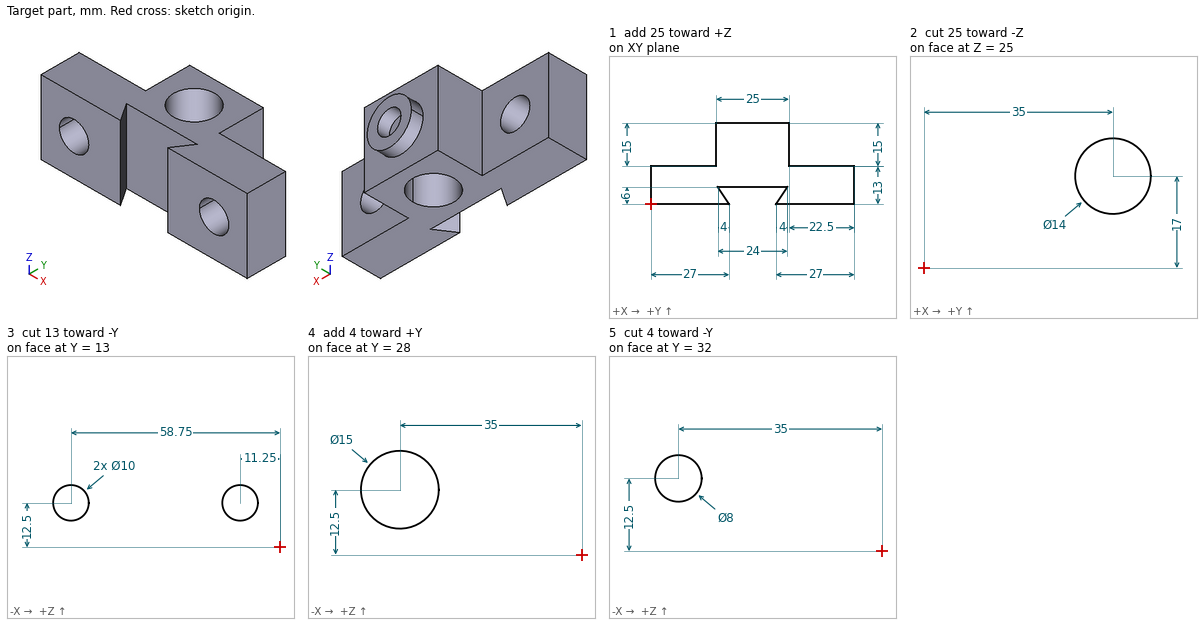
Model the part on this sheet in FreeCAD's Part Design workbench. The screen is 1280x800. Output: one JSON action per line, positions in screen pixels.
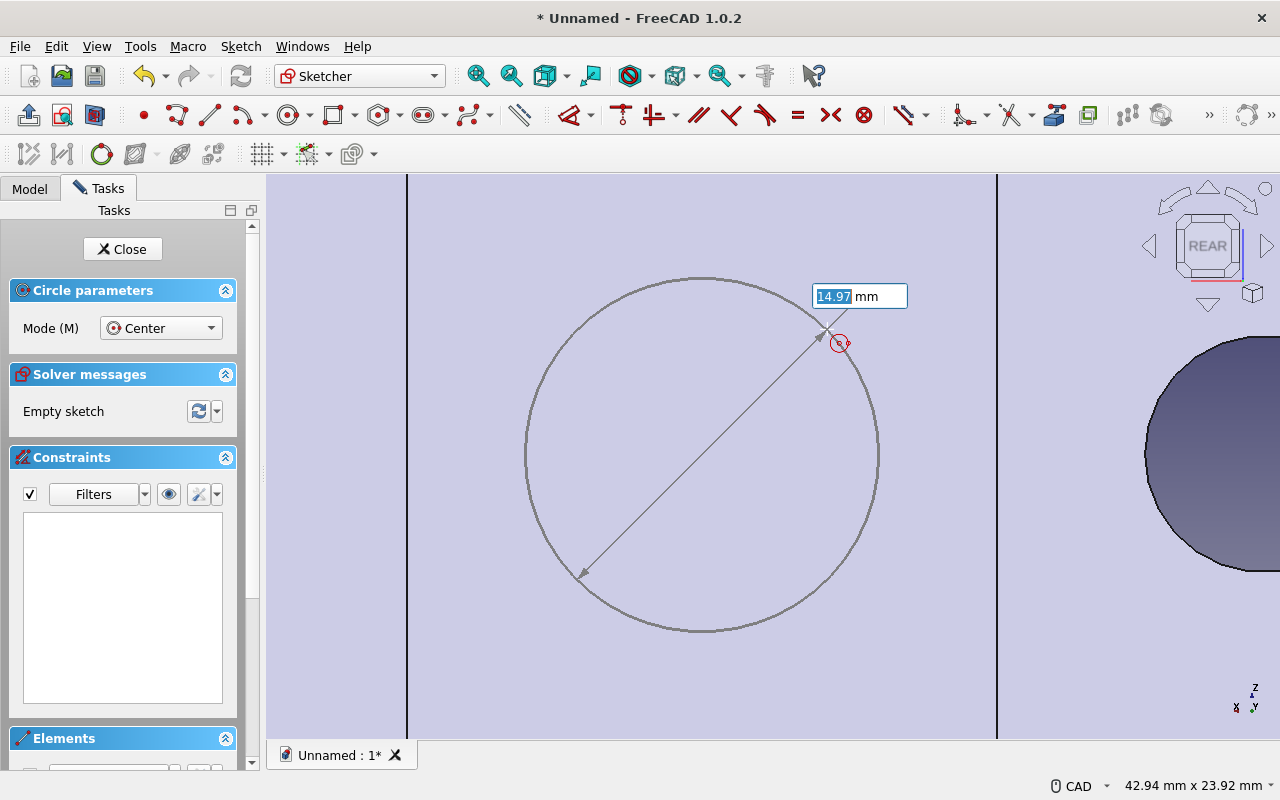
{"action": "type", "text": "15"}
{"action": "key", "text": "Return"}
{"action": "key", "text": "Escape"}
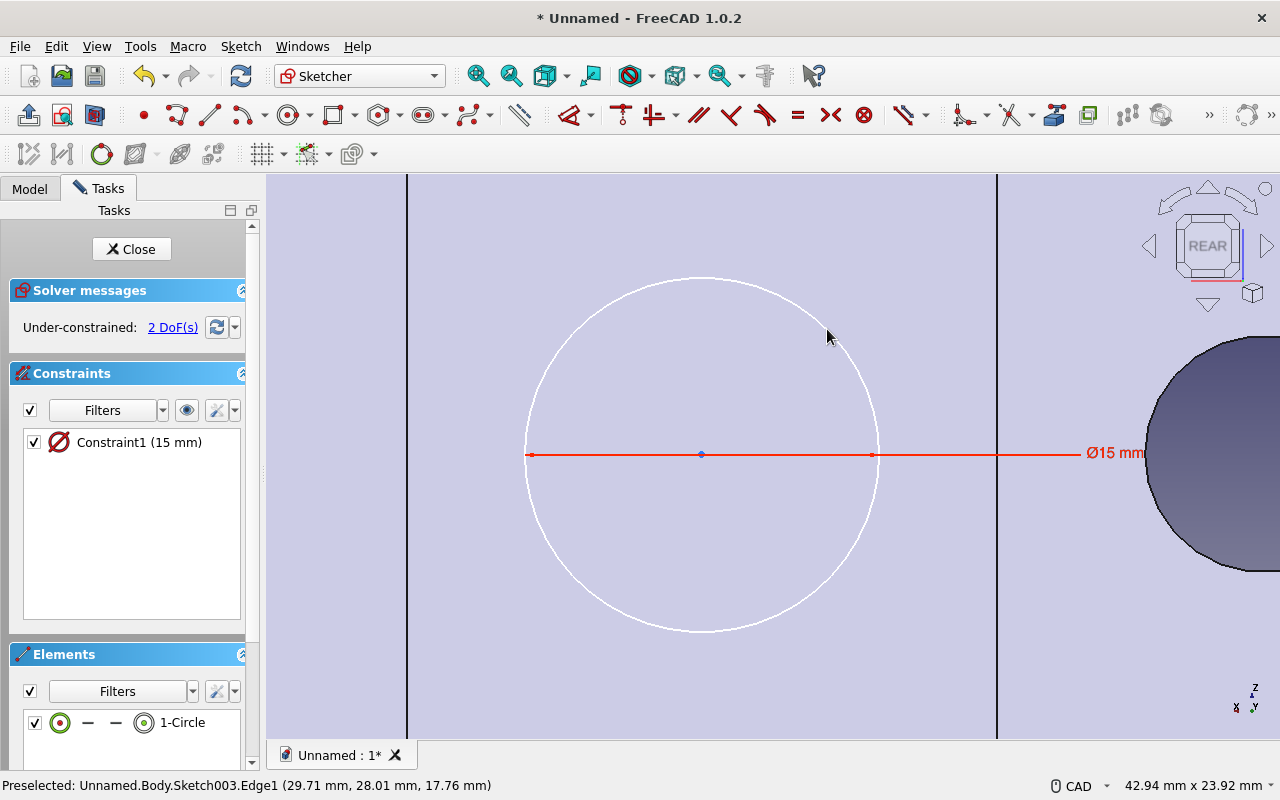
{"action": "left_click", "coordinate": [568, 116]}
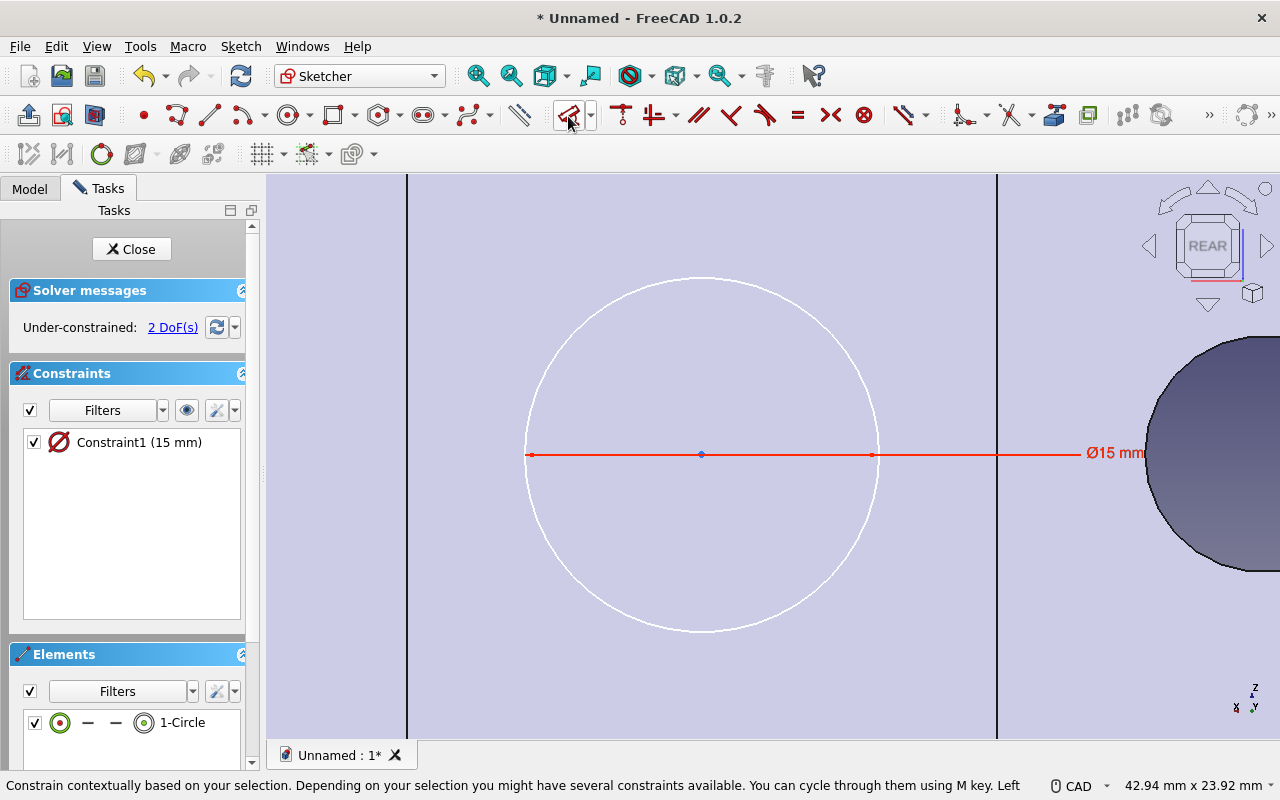
{"action": "left_click", "coordinate": [702, 455]}
{"action": "left_click", "coordinate": [908, 421]}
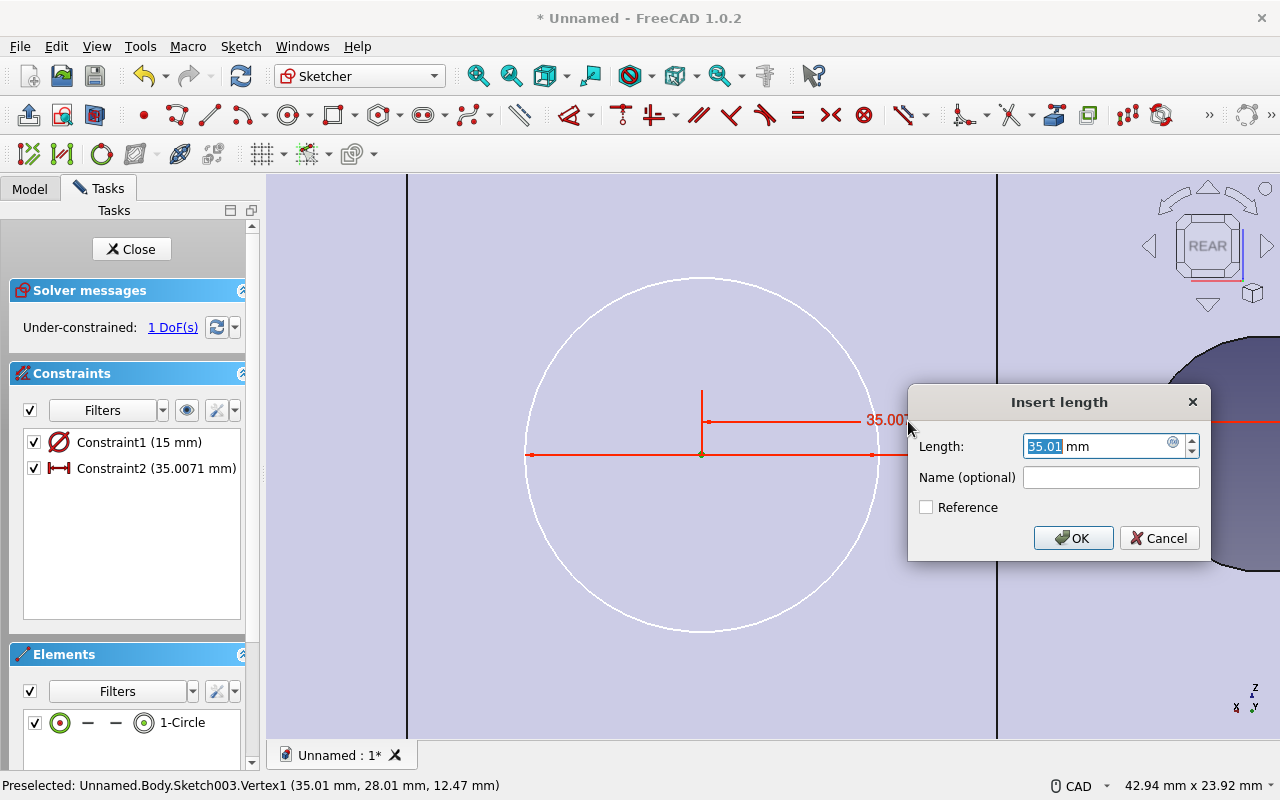
{"action": "type", "text": "35"}
{"action": "key", "text": "Return"}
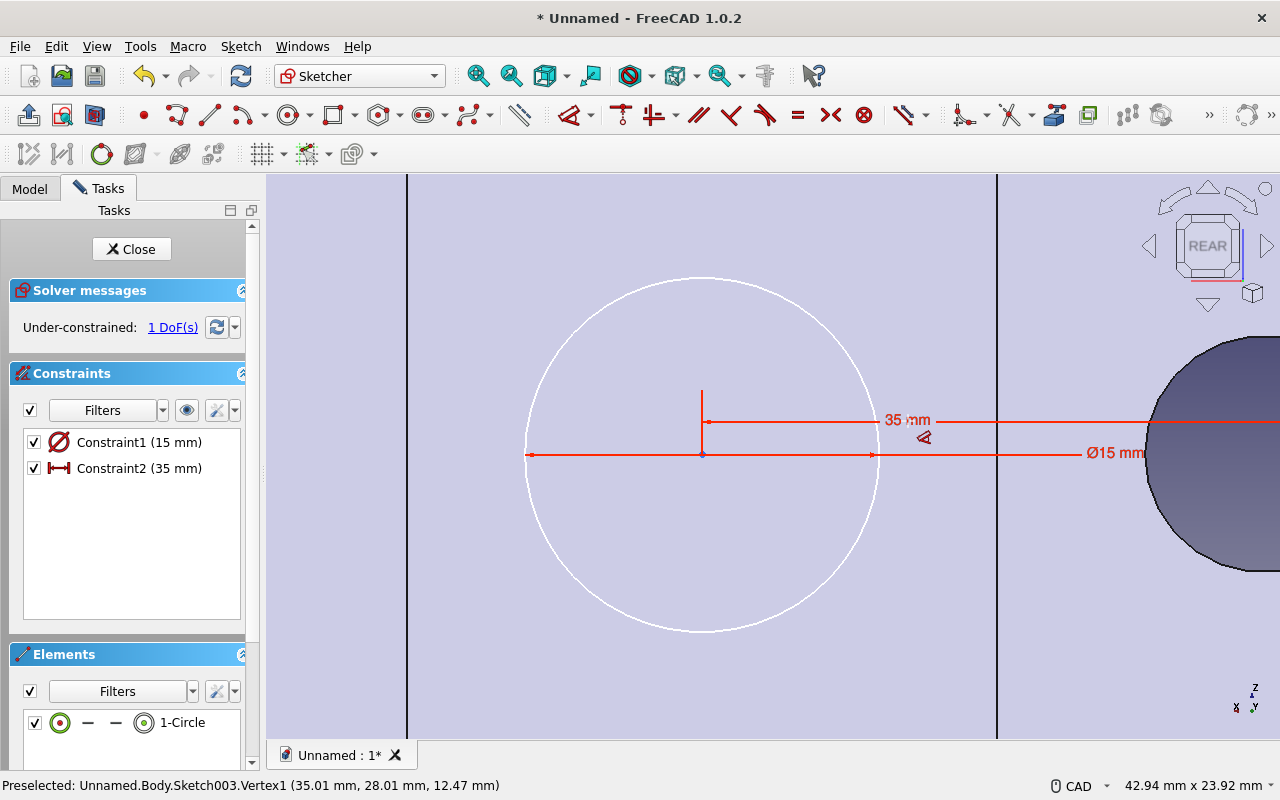
{"action": "left_click", "coordinate": [702, 455]}
{"action": "left_click", "coordinate": [668, 583]}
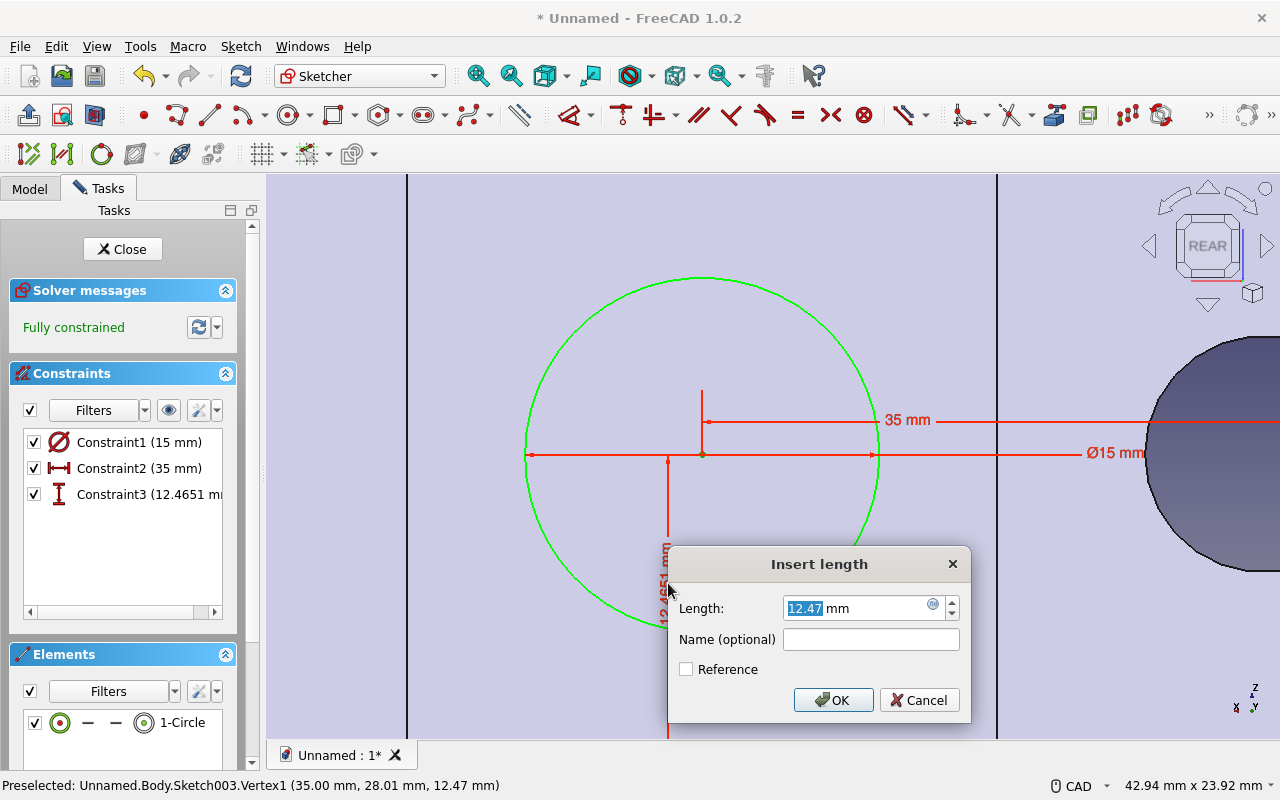
{"action": "type", "text": "12.5"}
{"action": "key", "text": "Return"}
{"action": "key", "text": "Escape"}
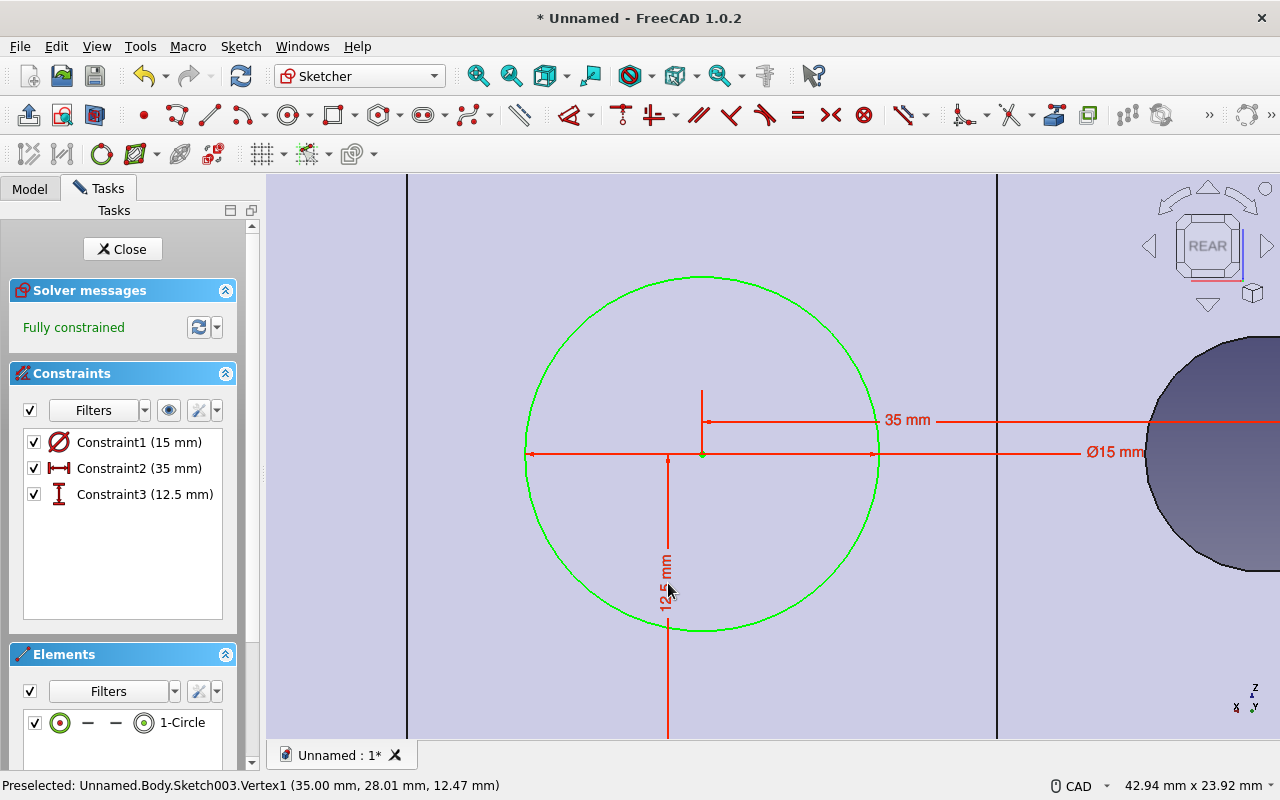
{"action": "left_click", "coordinate": [123, 249]}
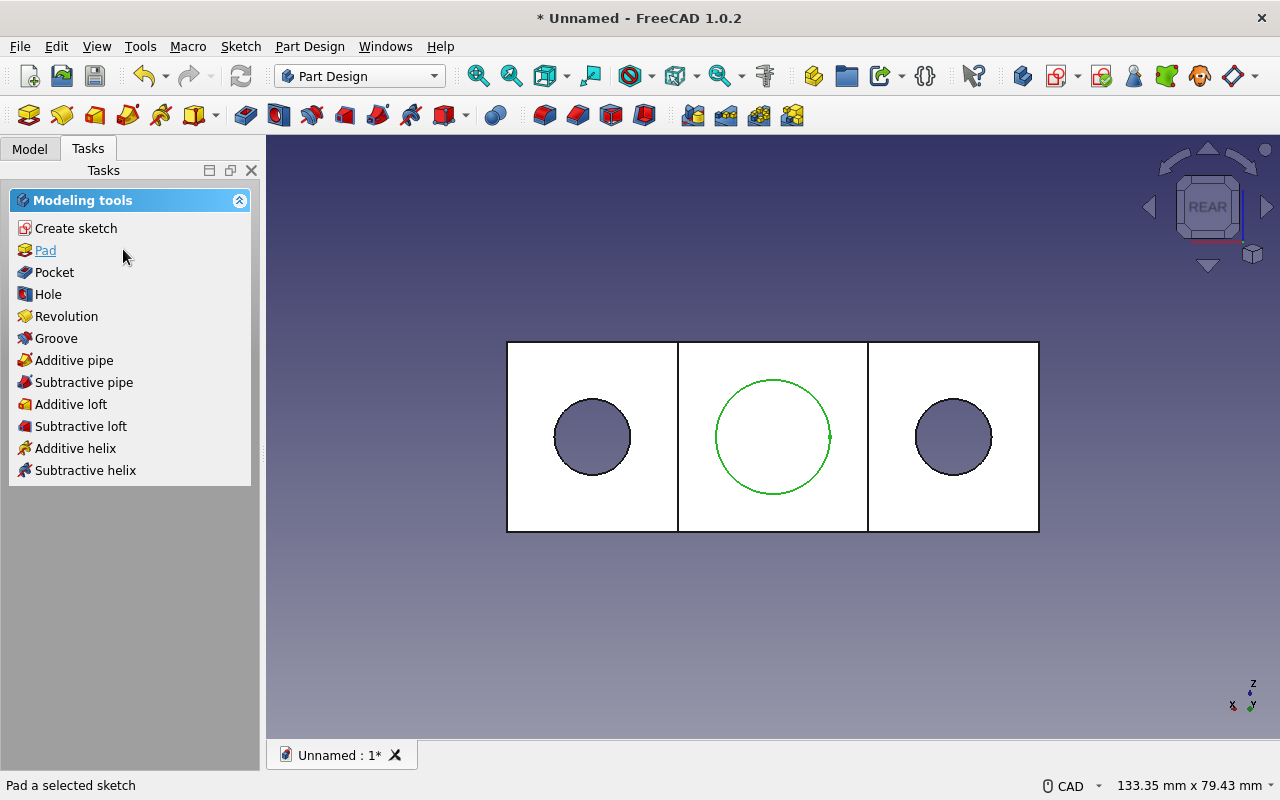
{"action": "left_click", "coordinate": [29, 116]}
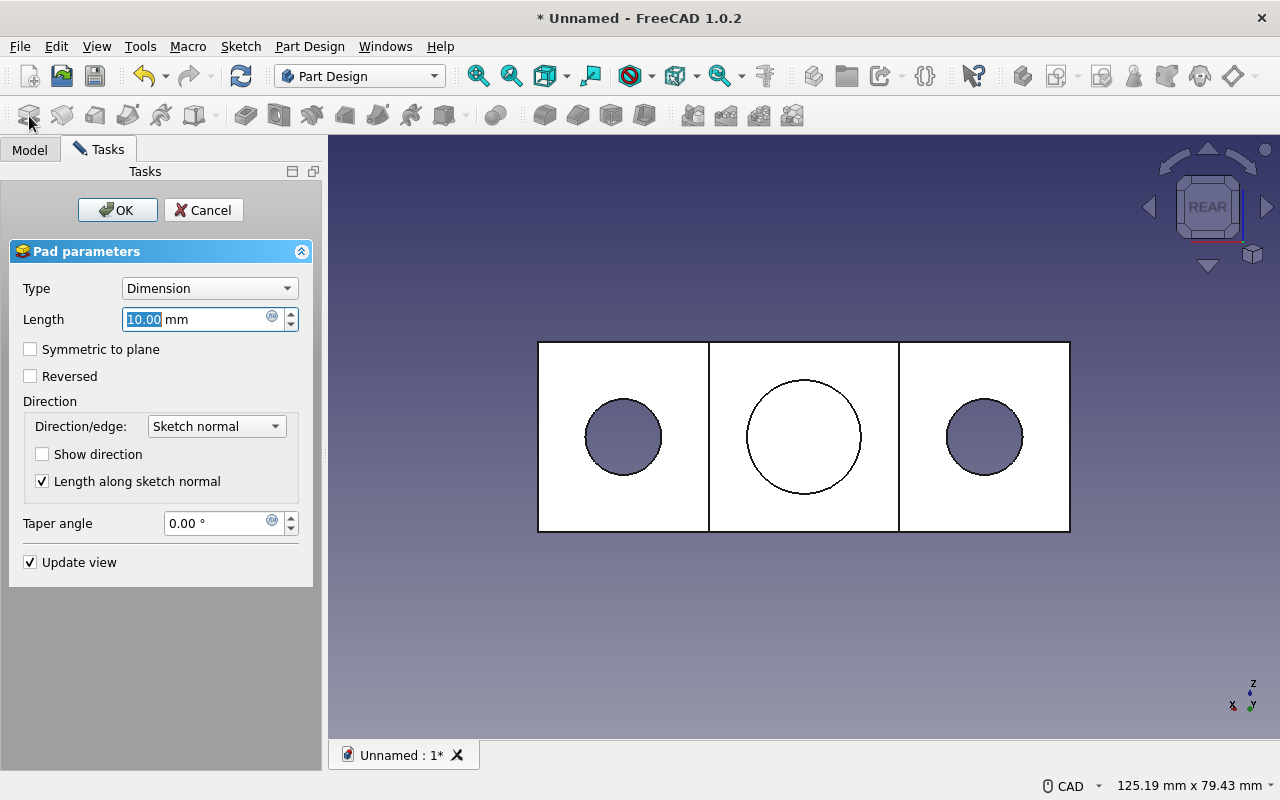
{"action": "type", "text": "4"}
{"action": "key", "text": "Tab"}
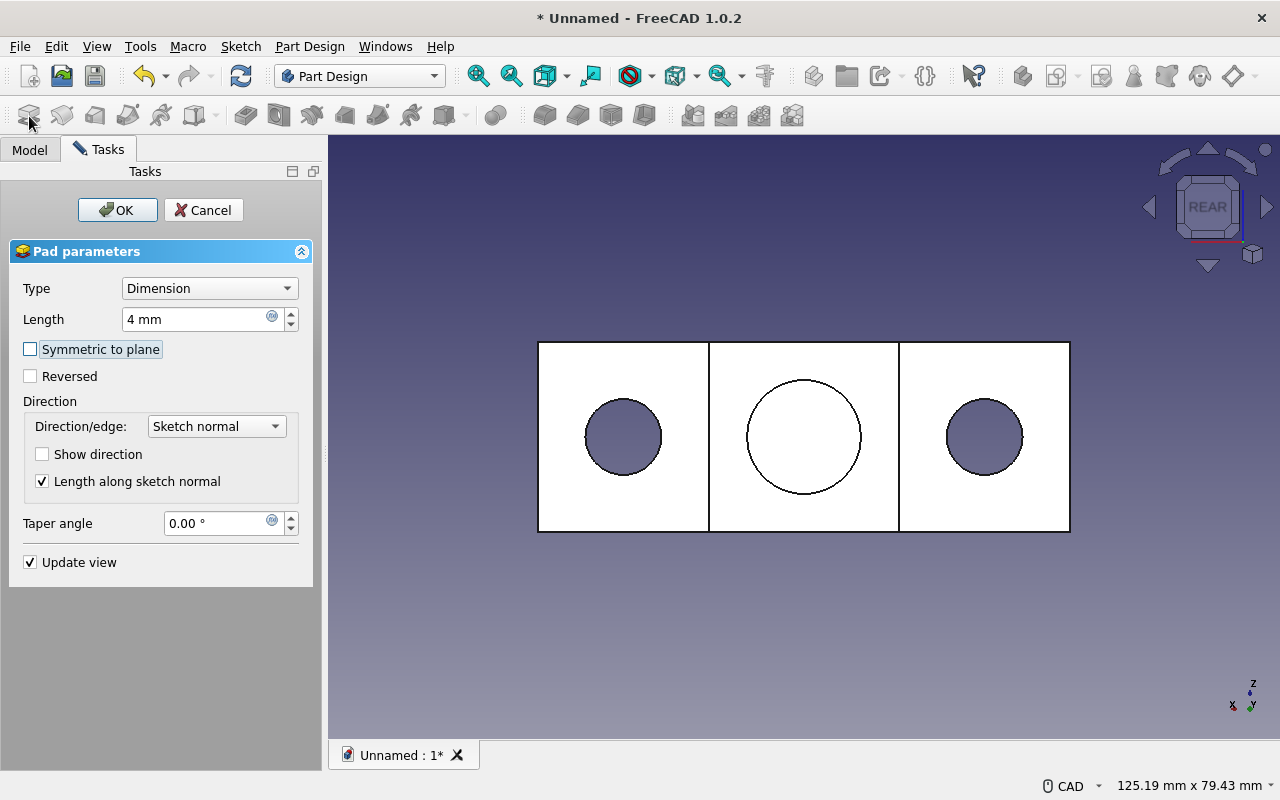
{"action": "left_click", "coordinate": [118, 210]}